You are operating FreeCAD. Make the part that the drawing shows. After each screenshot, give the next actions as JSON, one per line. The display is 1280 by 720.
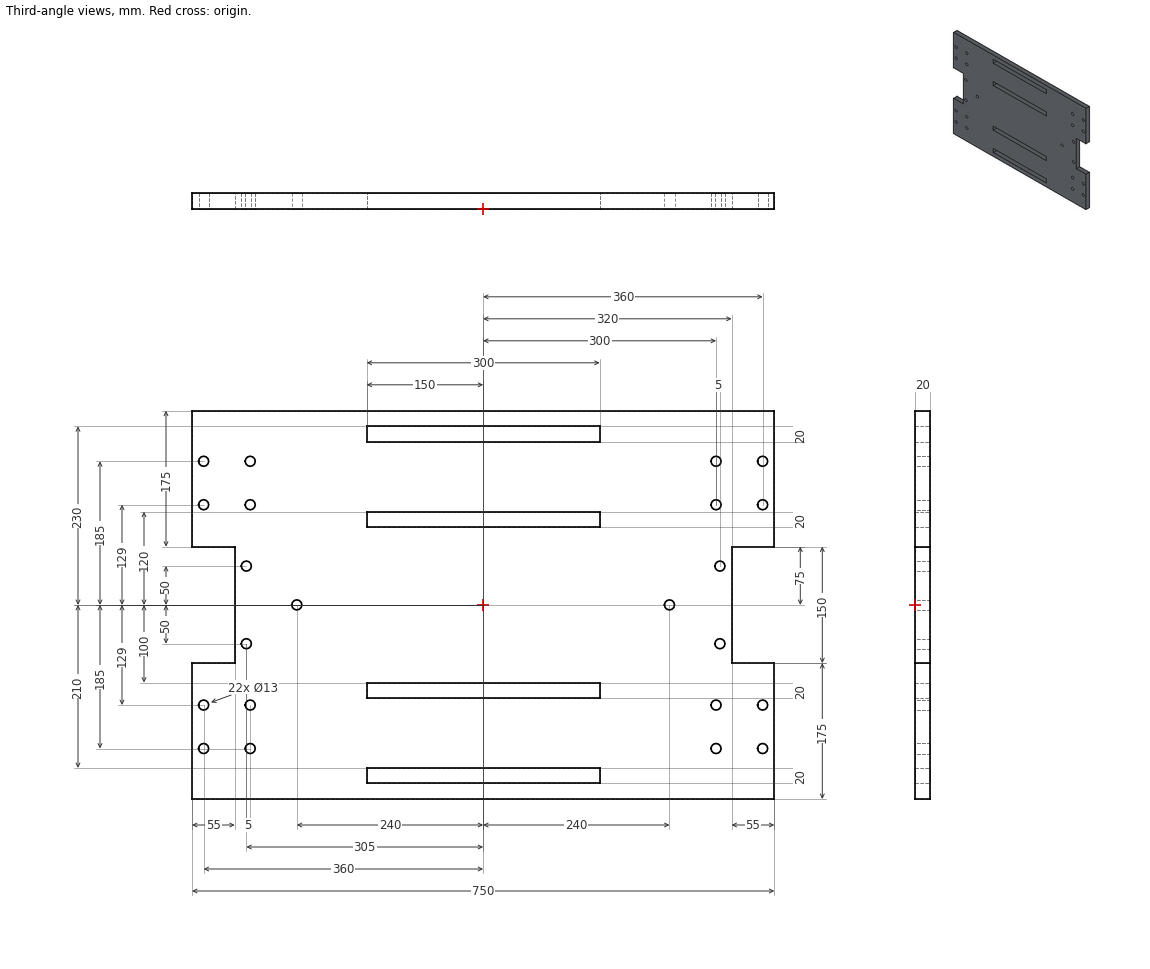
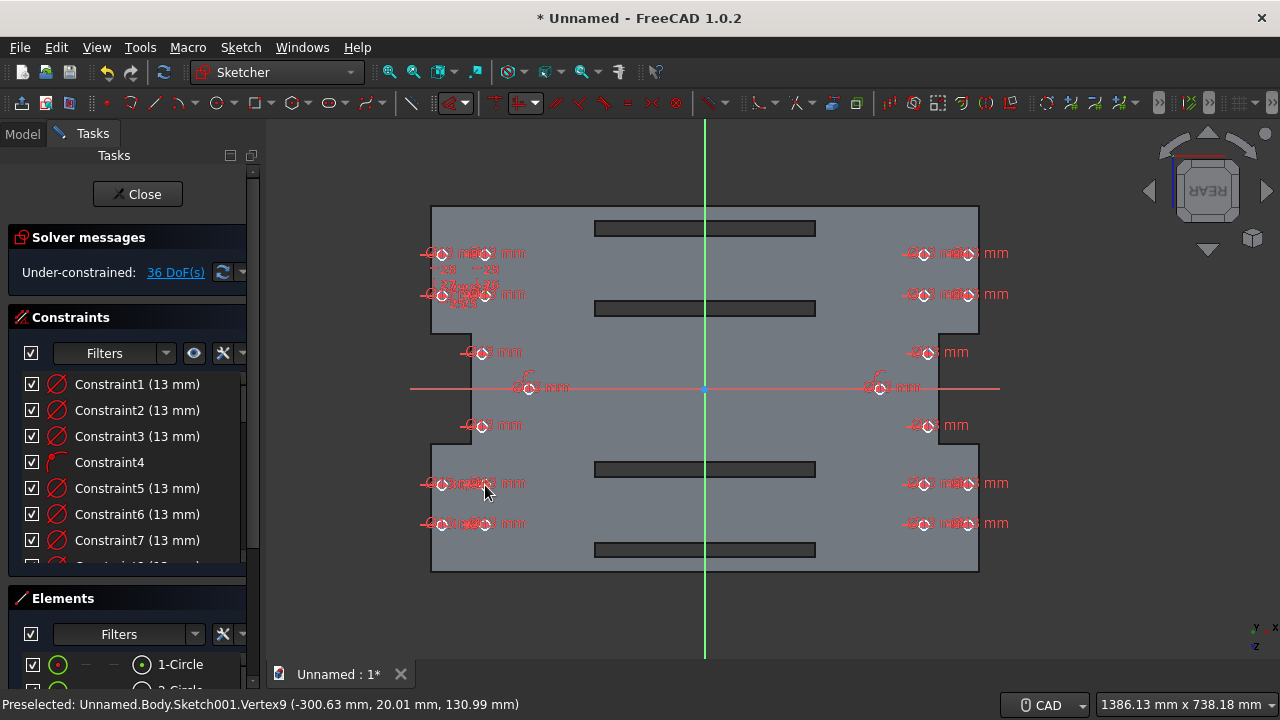
{"action": "left_click", "coordinate": [538, 104]}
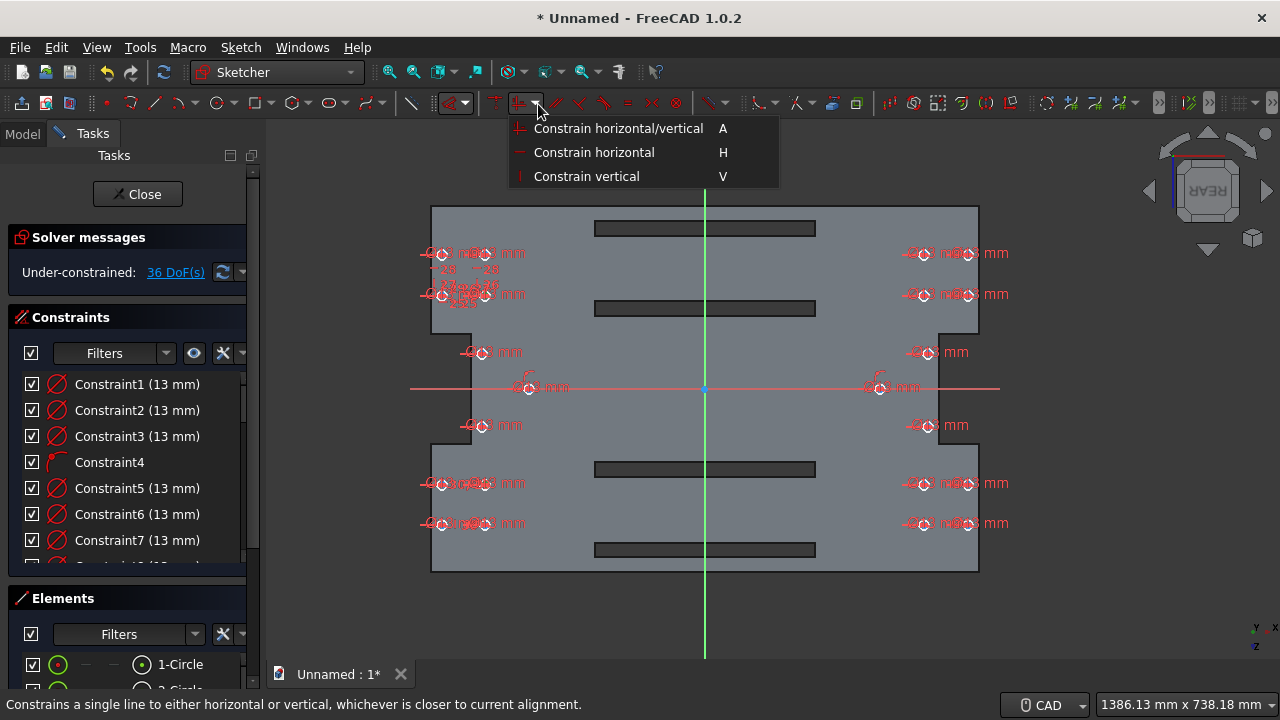
{"action": "left_click", "coordinate": [644, 176]}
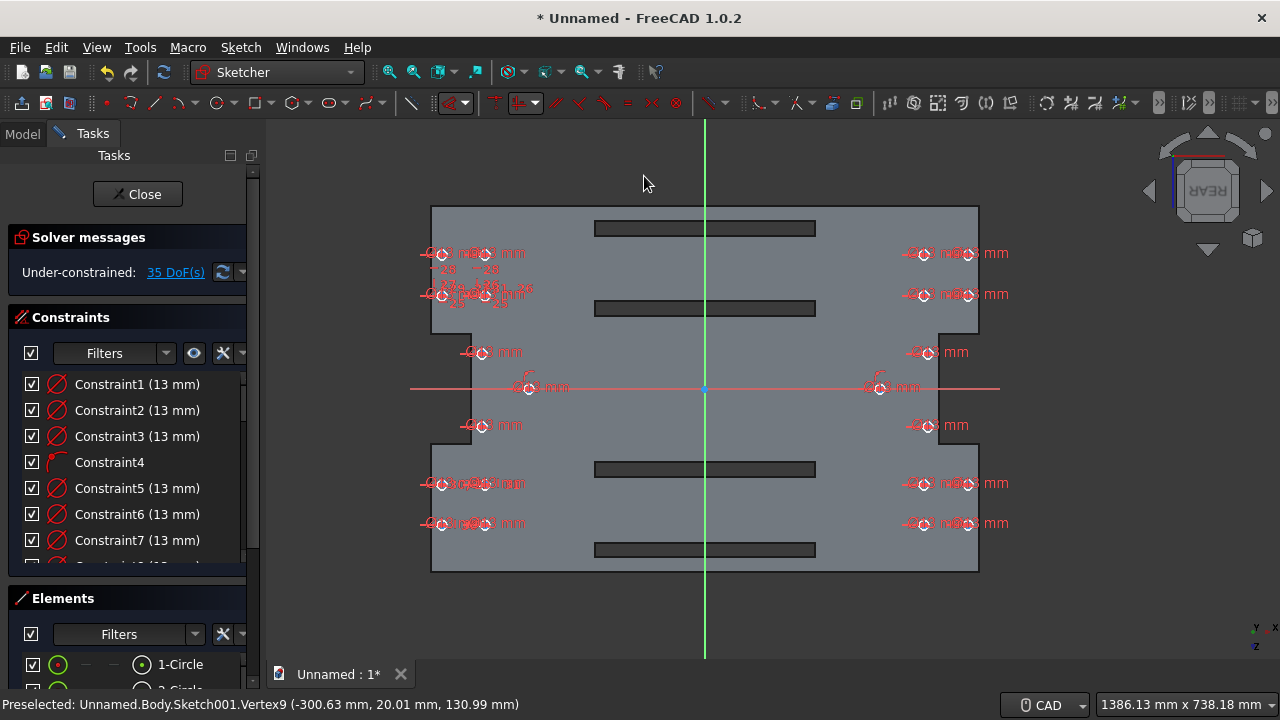
{"action": "left_click", "coordinate": [442, 485]}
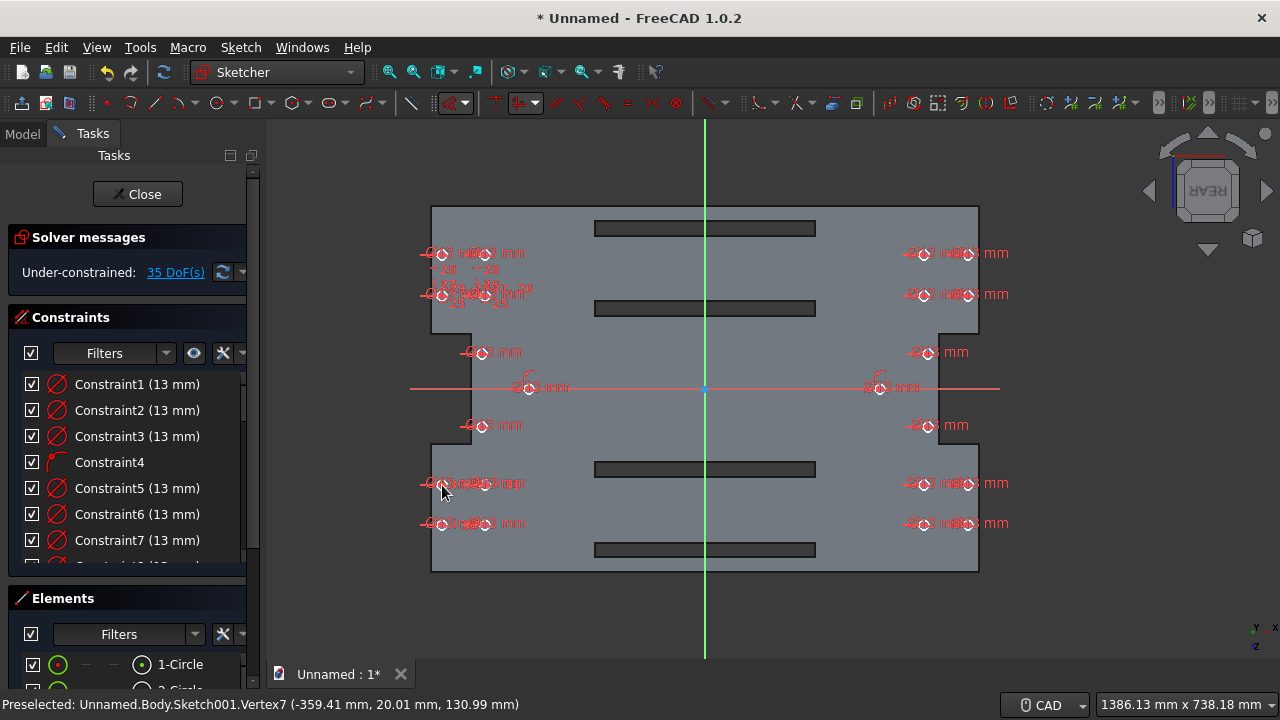
{"action": "left_click", "coordinate": [485, 485]}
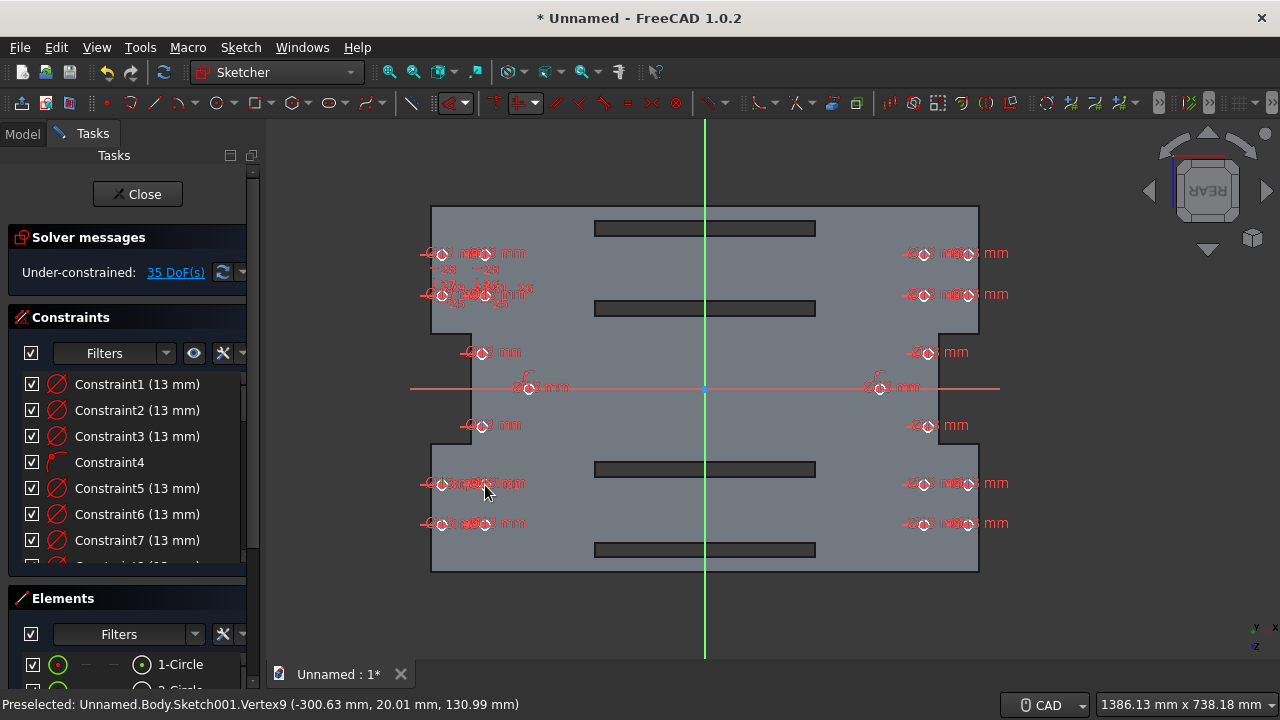
{"action": "left_click", "coordinate": [538, 104]}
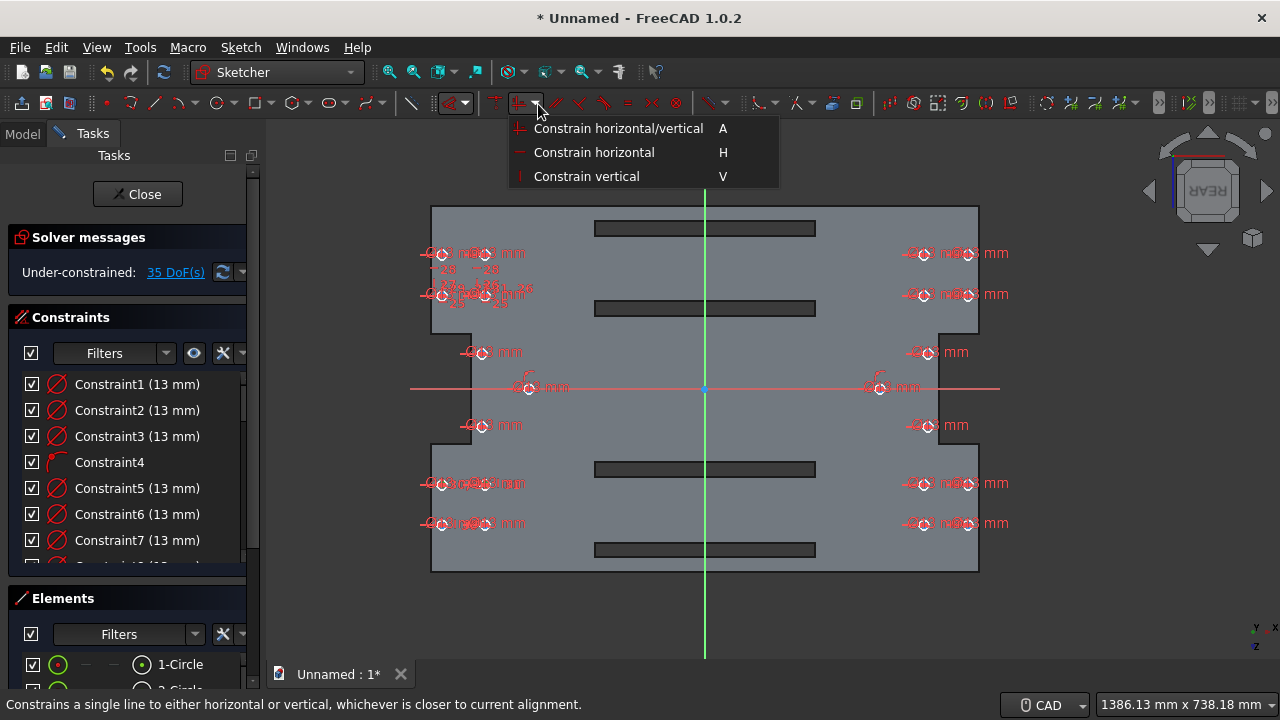
{"action": "left_click", "coordinate": [644, 152]}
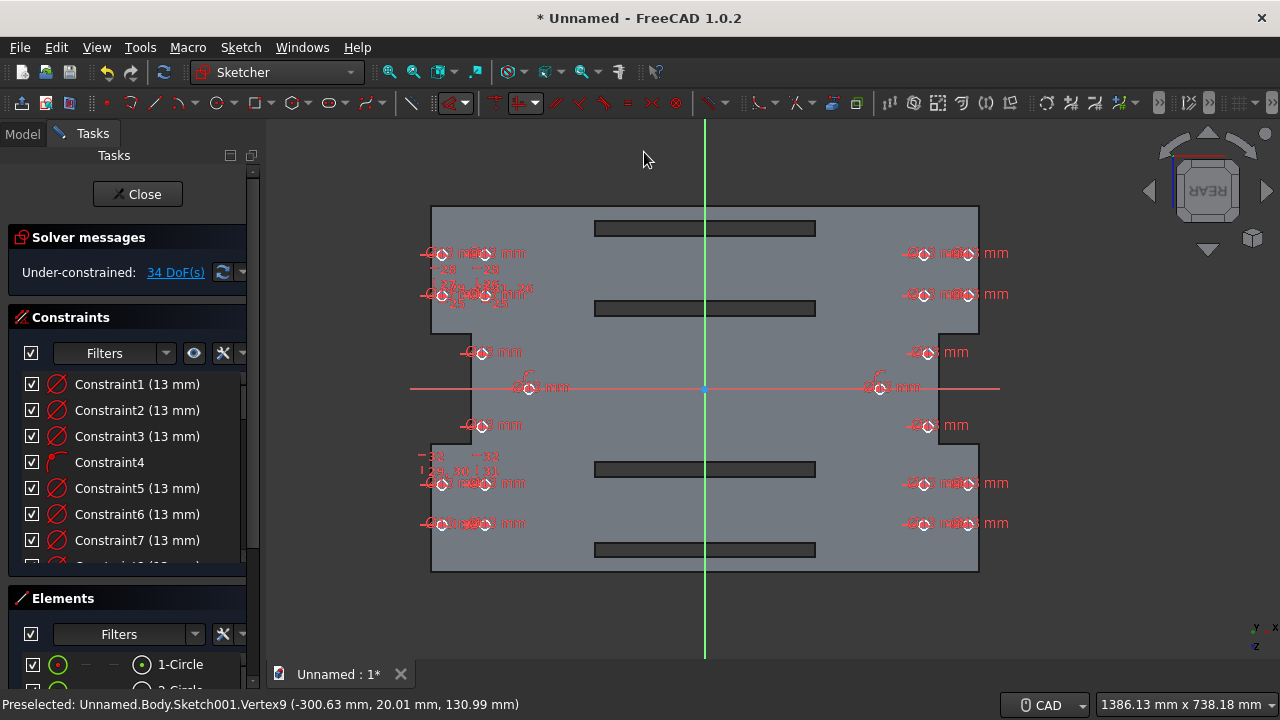
{"action": "left_click", "coordinate": [485, 485]}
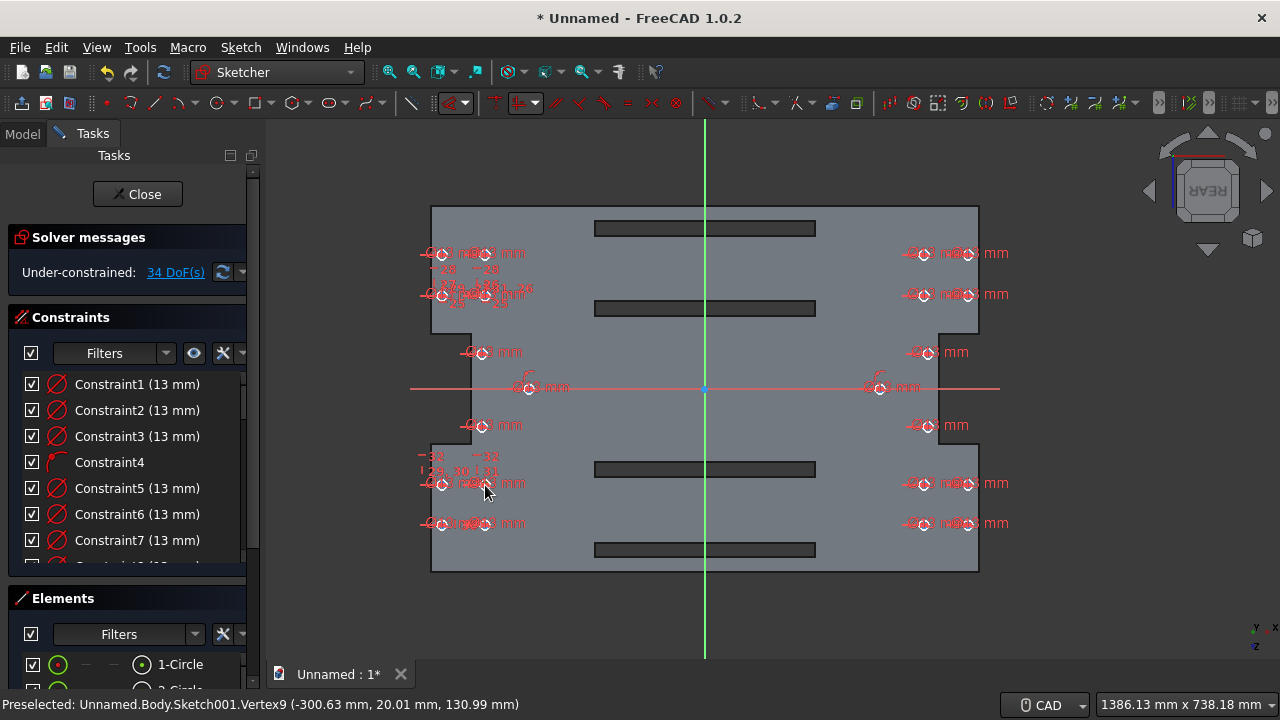
{"action": "left_click", "coordinate": [485, 525]}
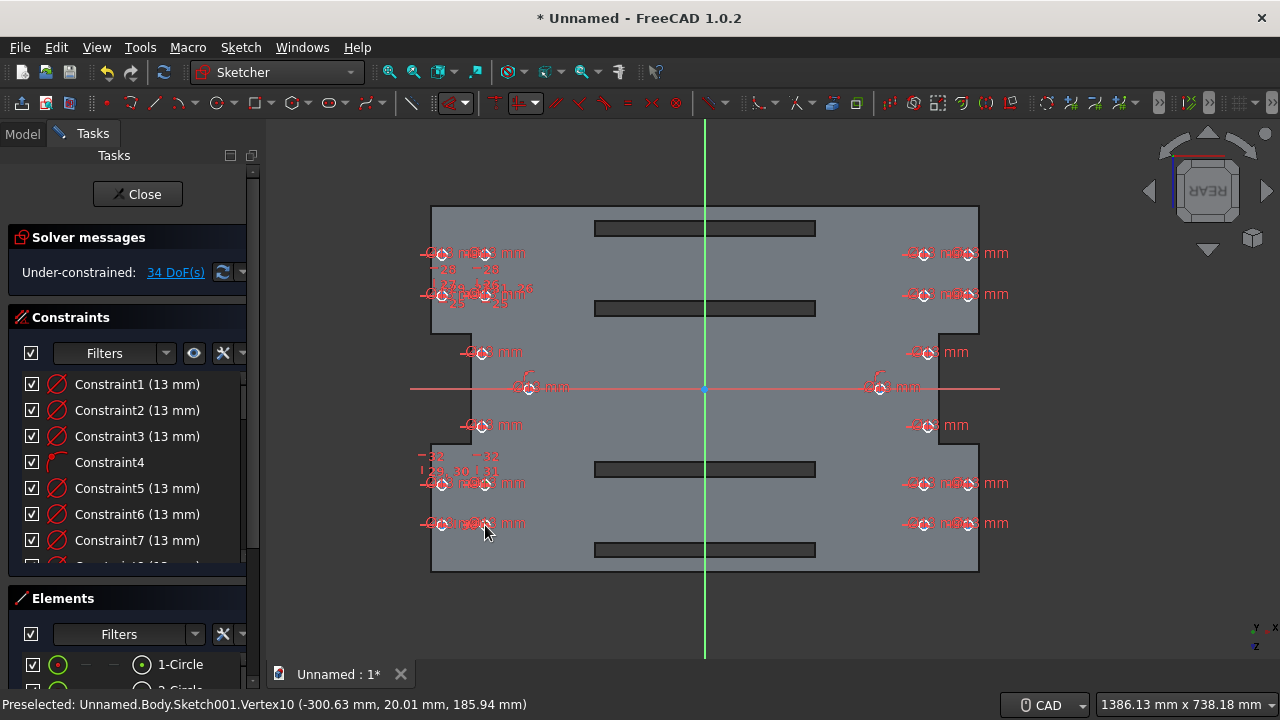
{"action": "key", "text": "v"}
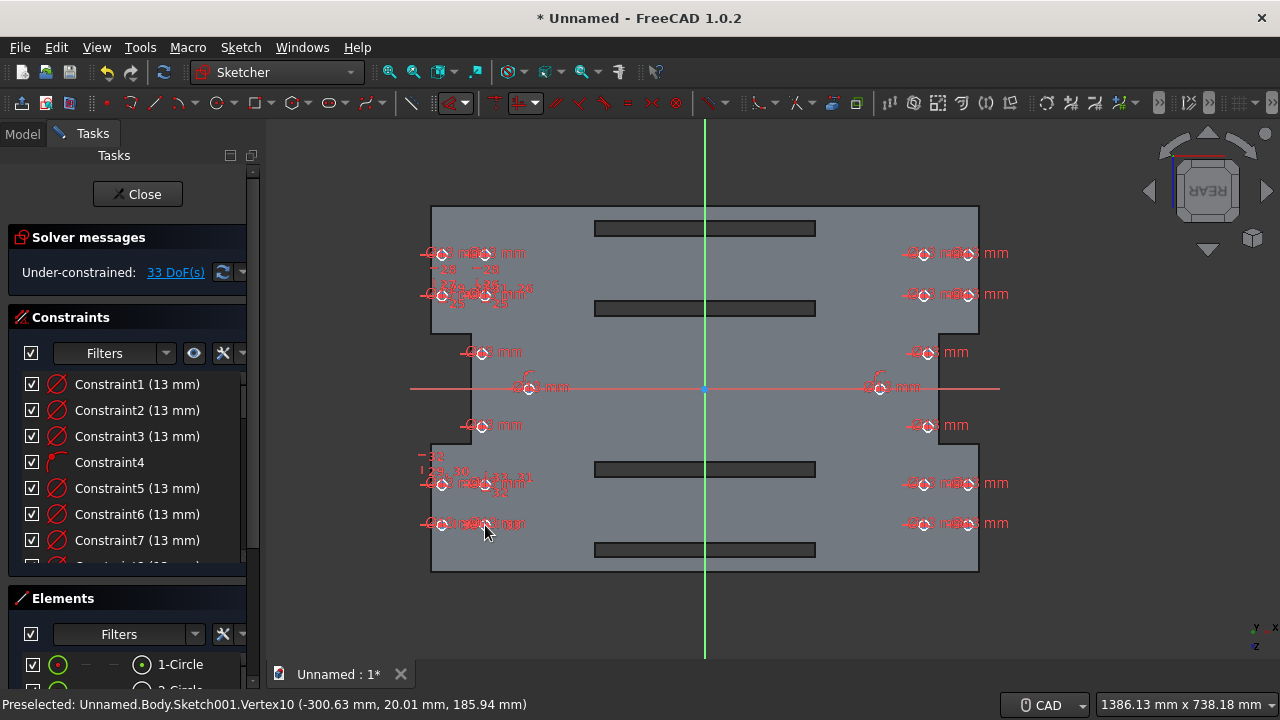
{"action": "left_click", "coordinate": [442, 525]}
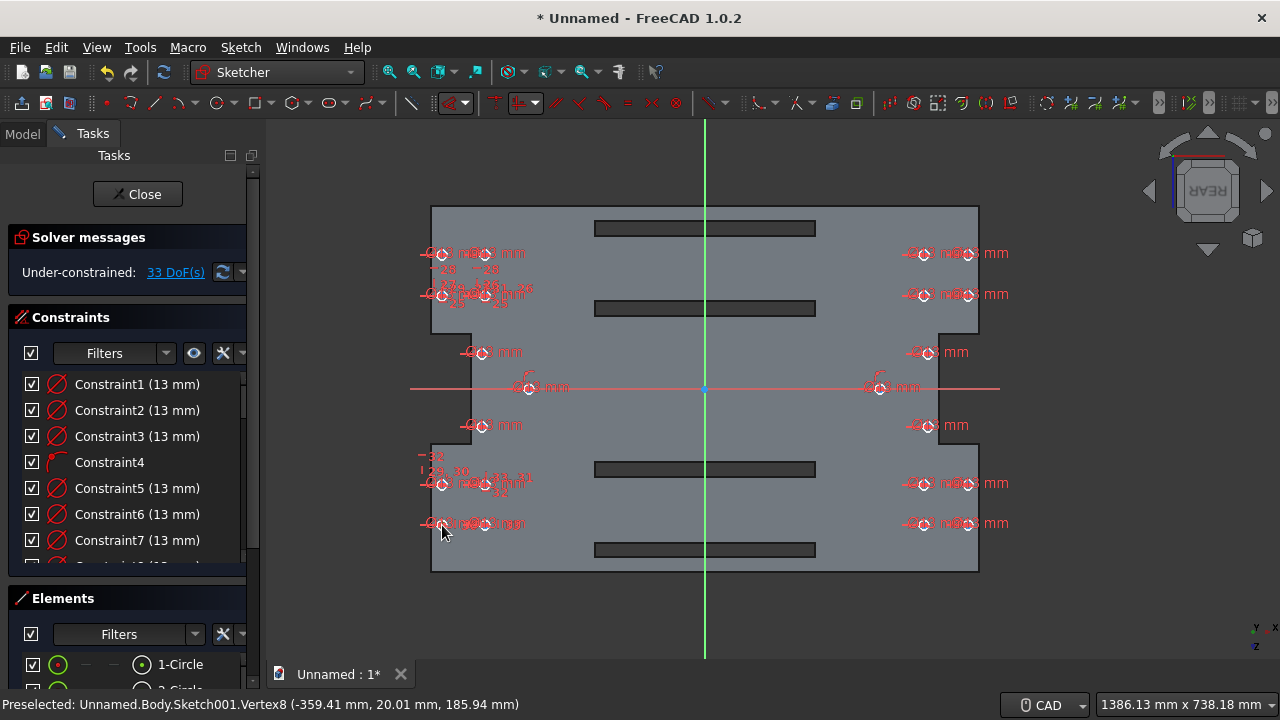
{"action": "left_click", "coordinate": [485, 525]}